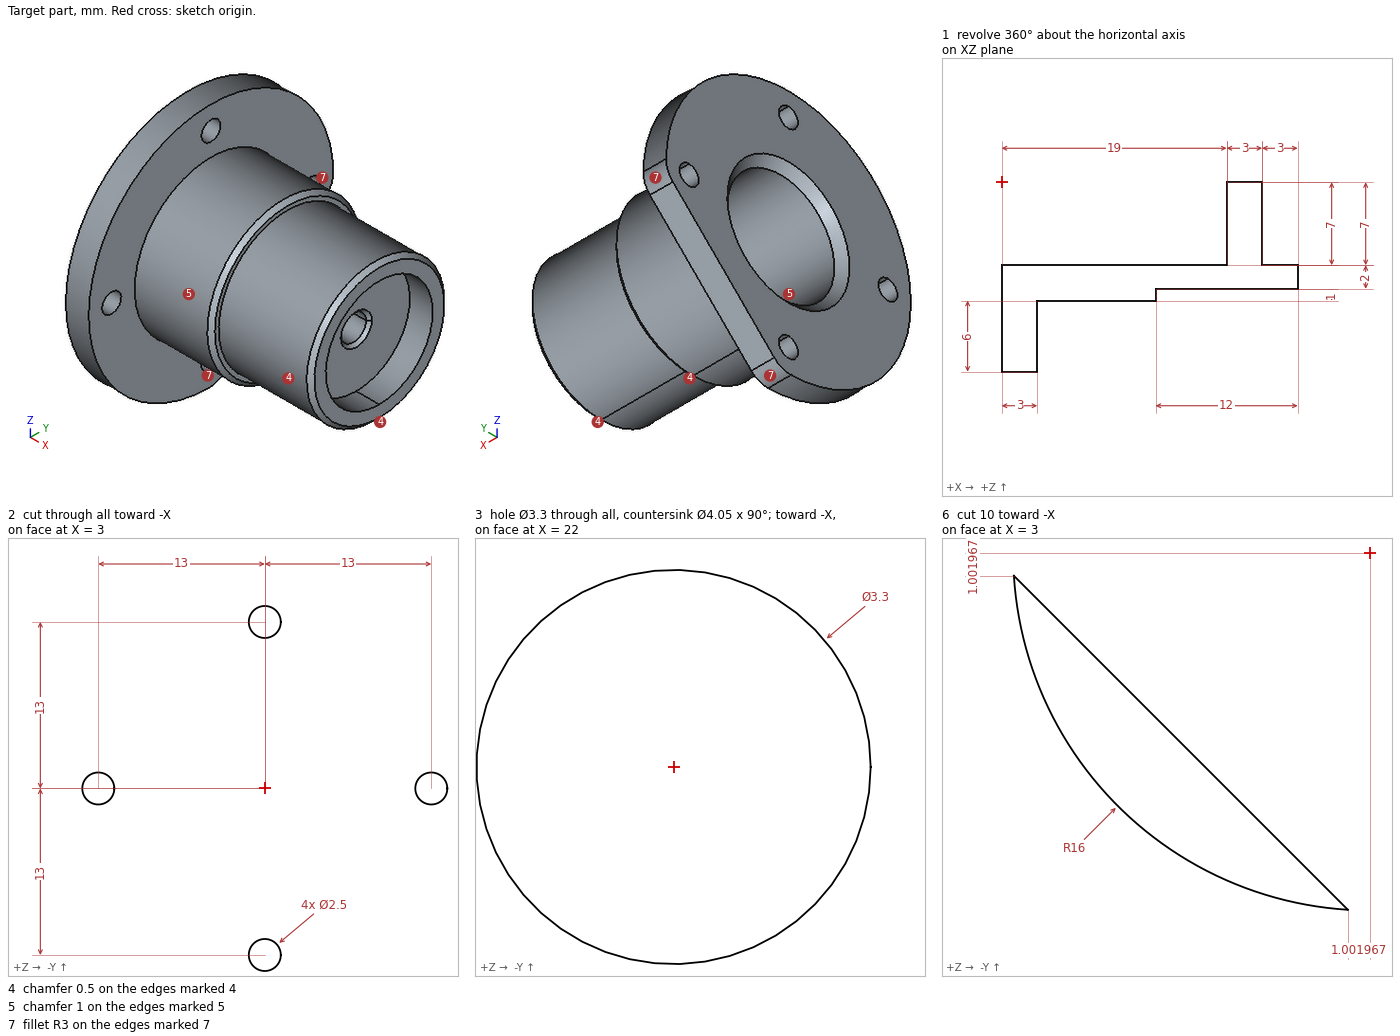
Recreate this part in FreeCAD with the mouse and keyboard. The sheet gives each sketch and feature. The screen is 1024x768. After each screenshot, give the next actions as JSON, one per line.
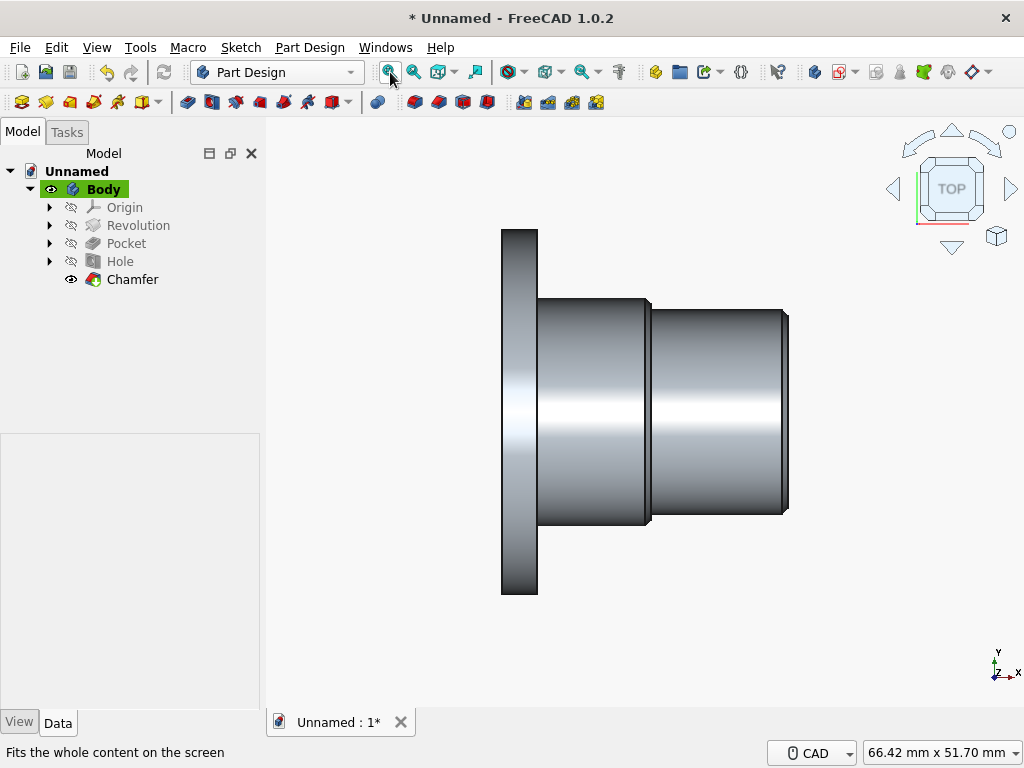
{"action": "key", "text": "0"}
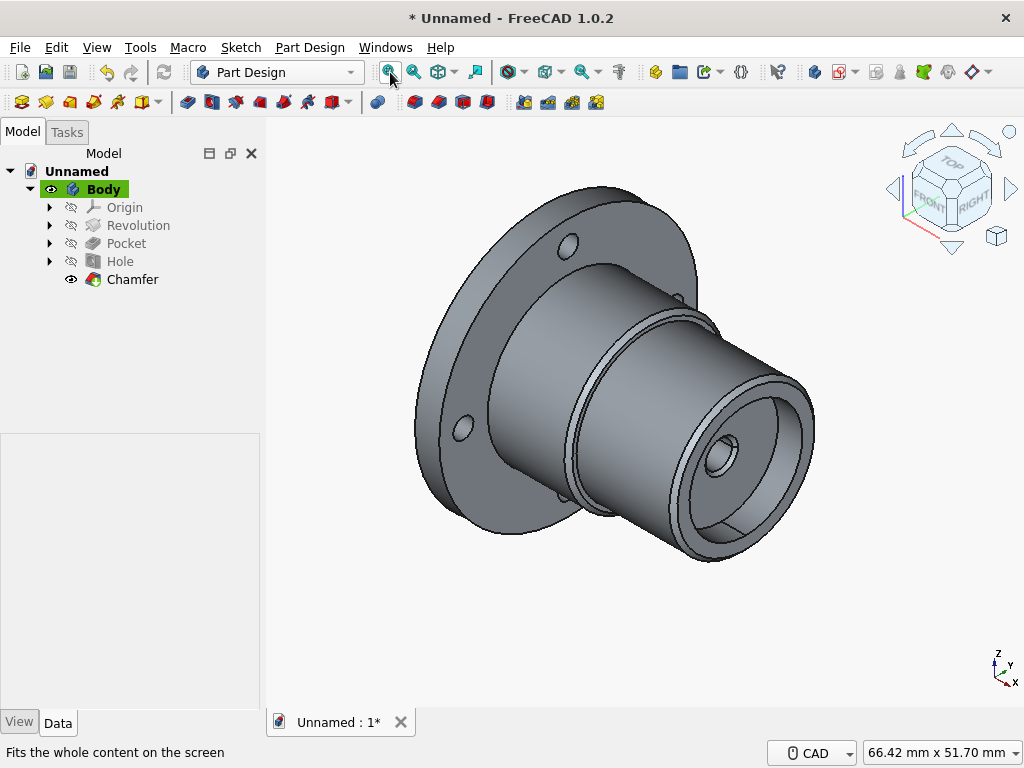
{"action": "key", "text": "1"}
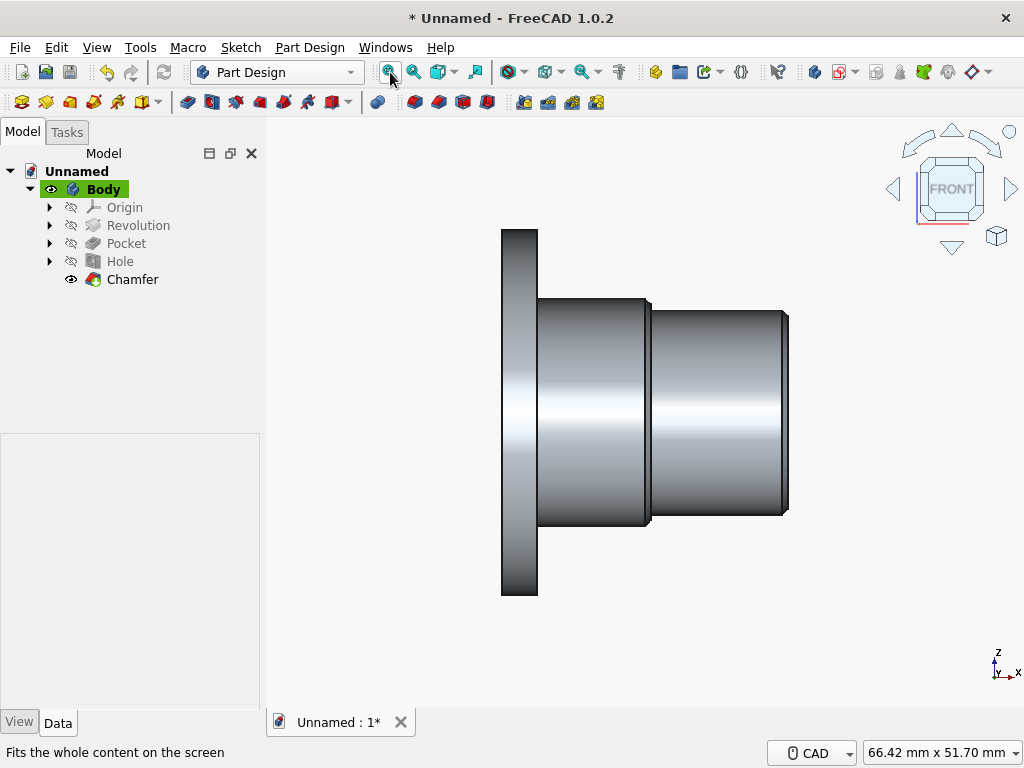
{"action": "key", "text": "3"}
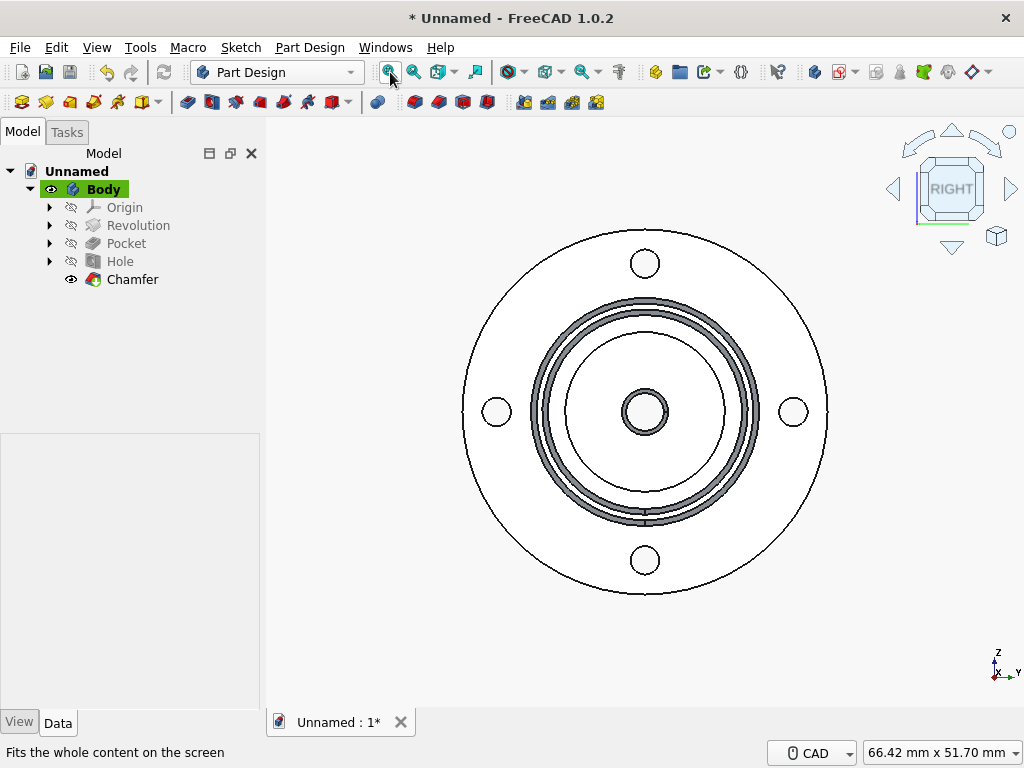
{"action": "key", "text": "5"}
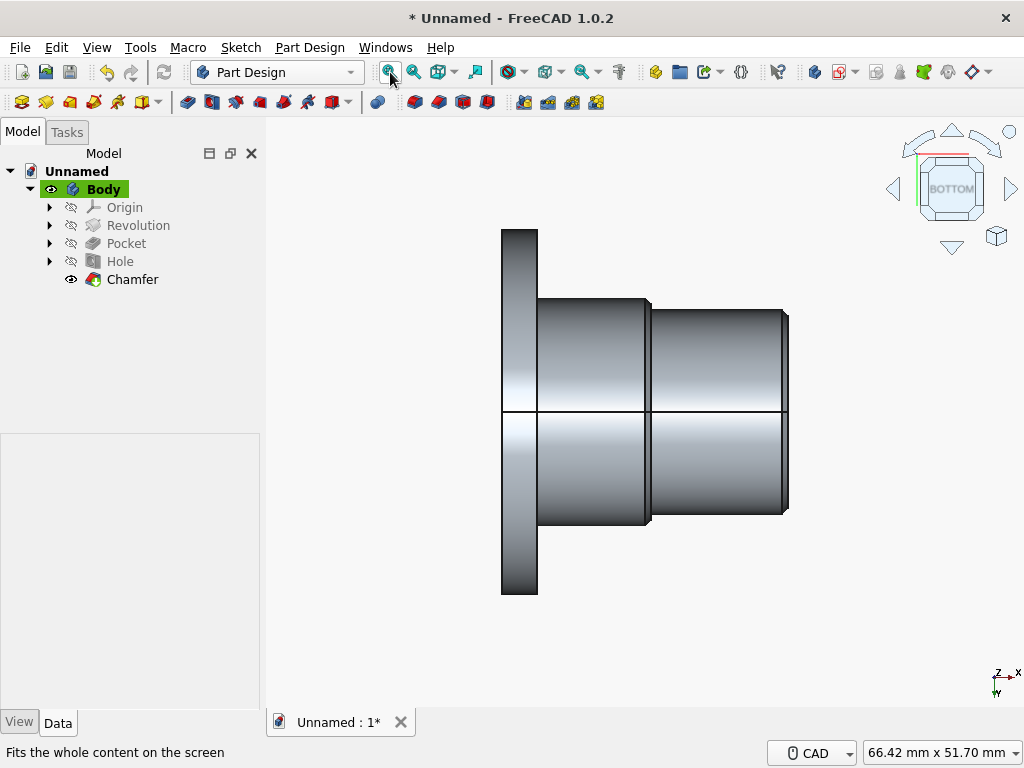
{"action": "key", "text": "4"}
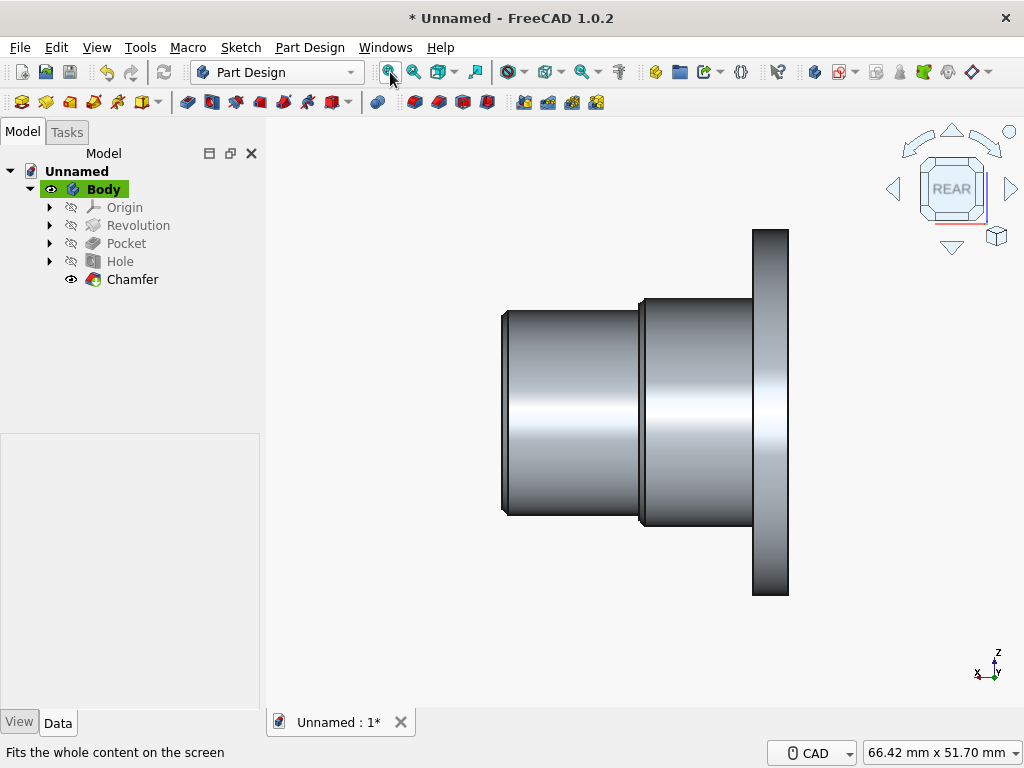
{"action": "key", "text": "6"}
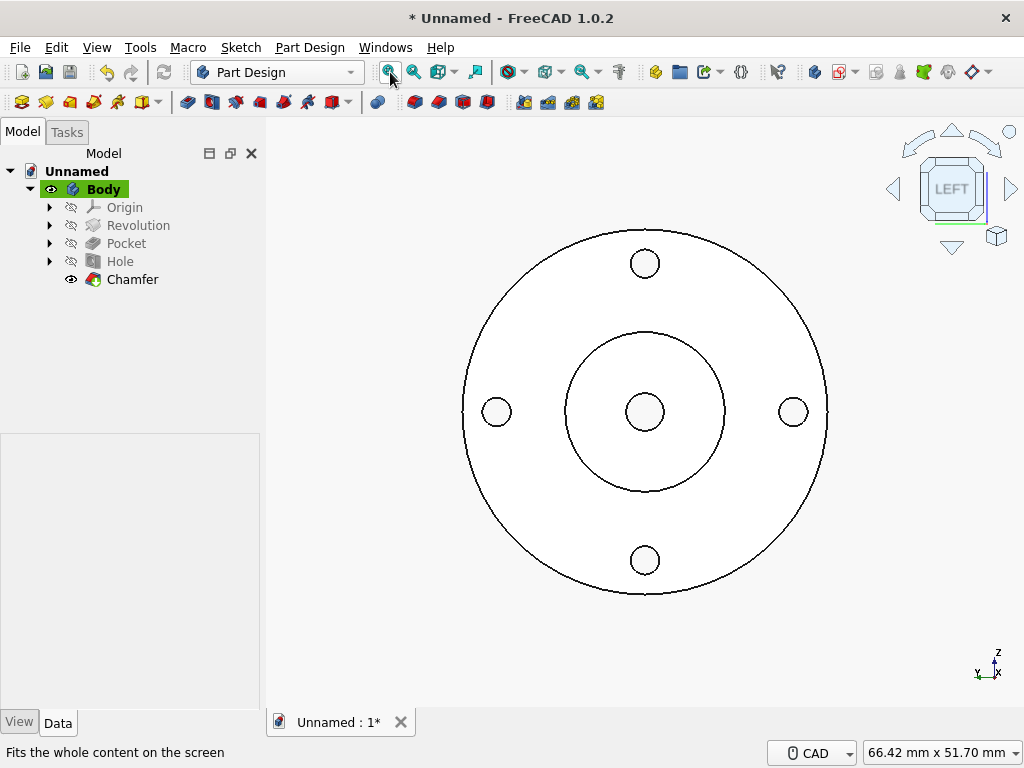
{"action": "left_click", "coordinate": [692, 346]}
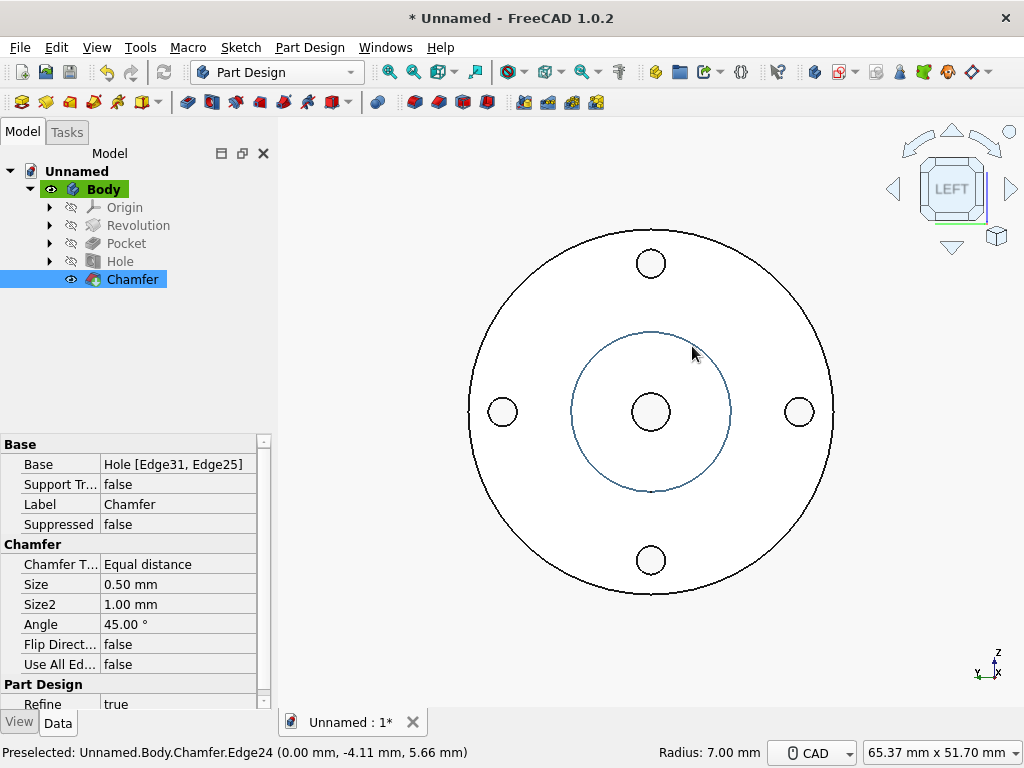
{"action": "left_click", "coordinate": [440, 102]}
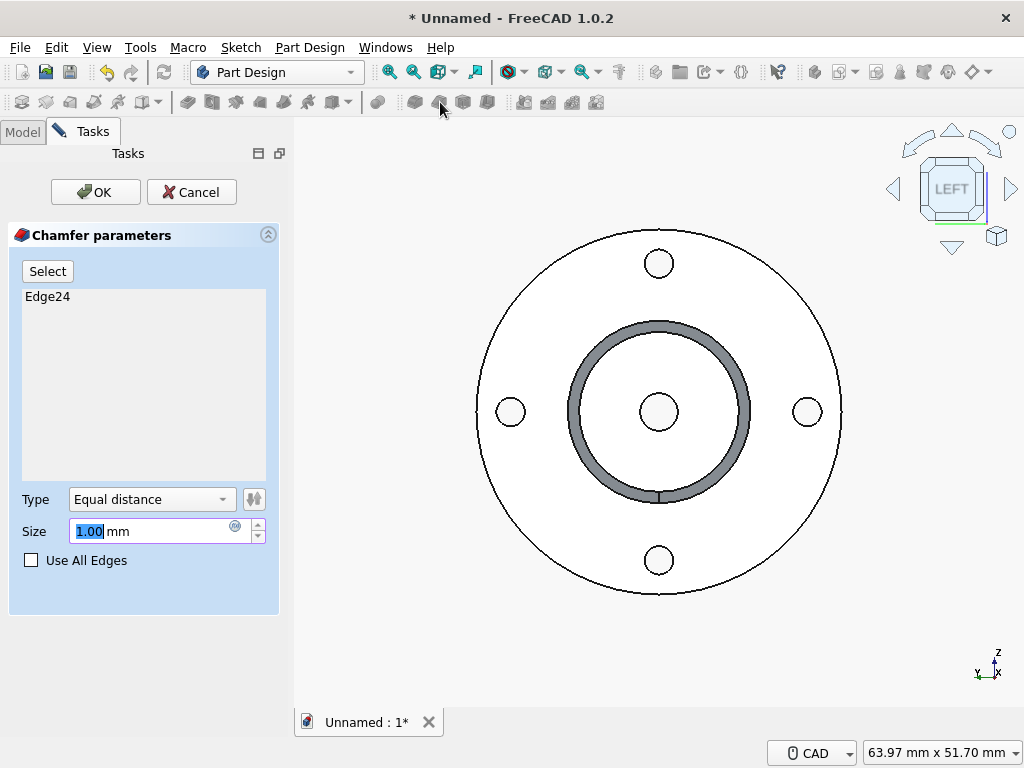
{"action": "type", "text": "1"}
{"action": "key", "text": "Tab"}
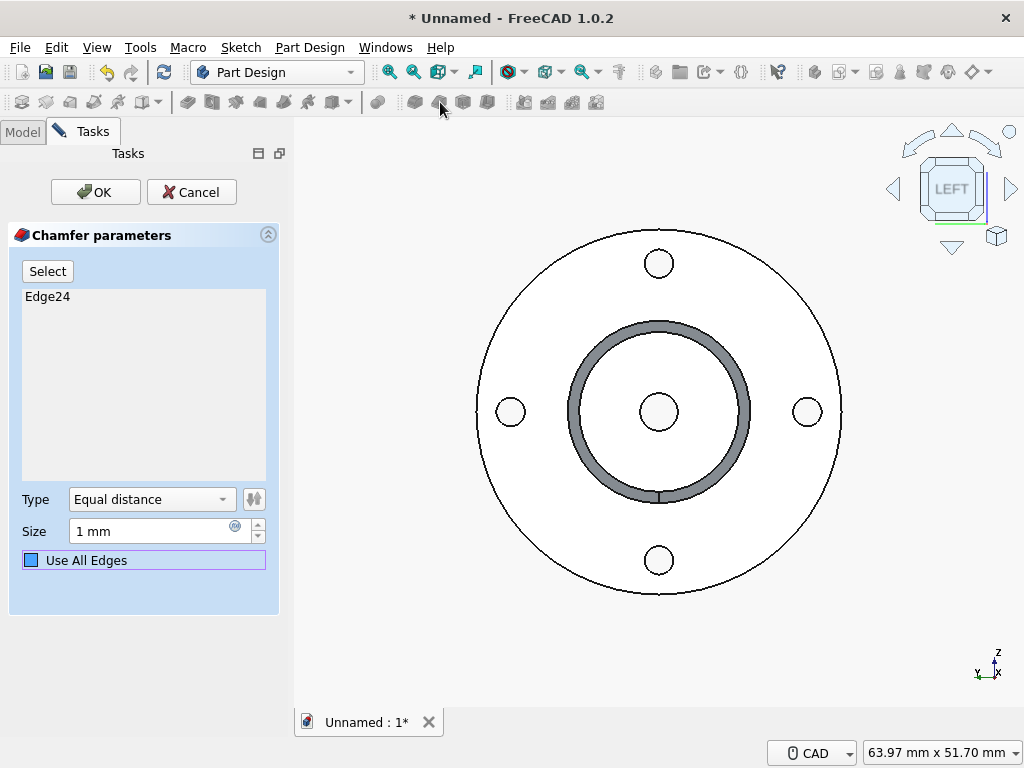
{"action": "left_click", "coordinate": [96, 192]}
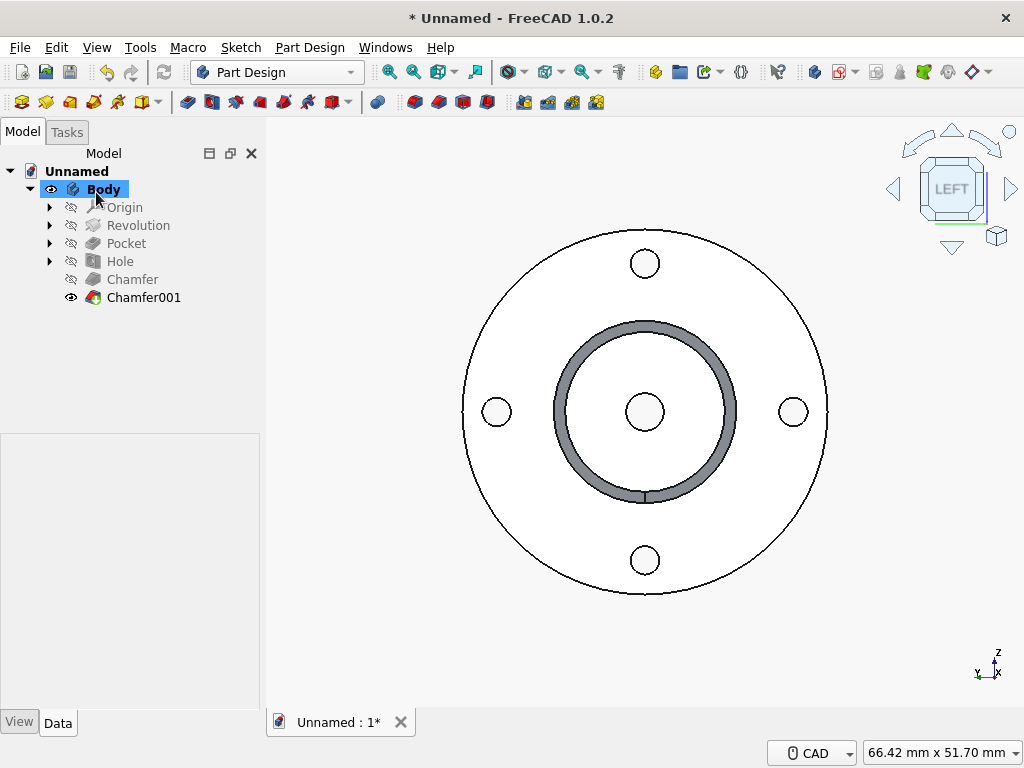
{"action": "key", "text": "0"}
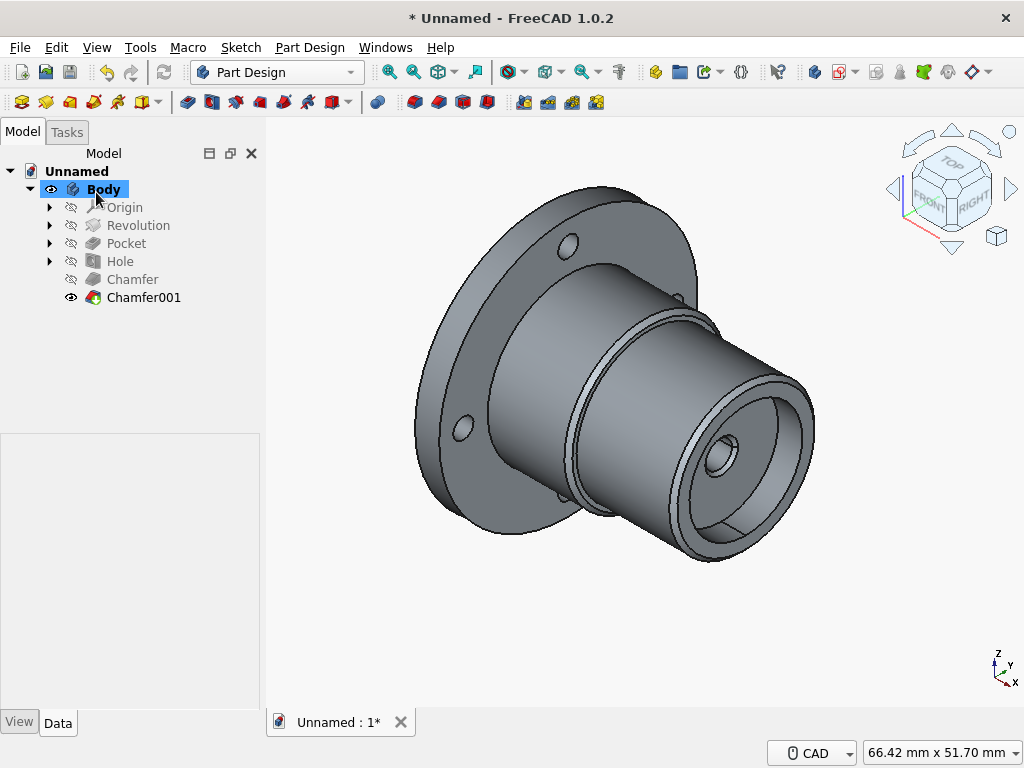
{"action": "left_click", "coordinate": [495, 324]}